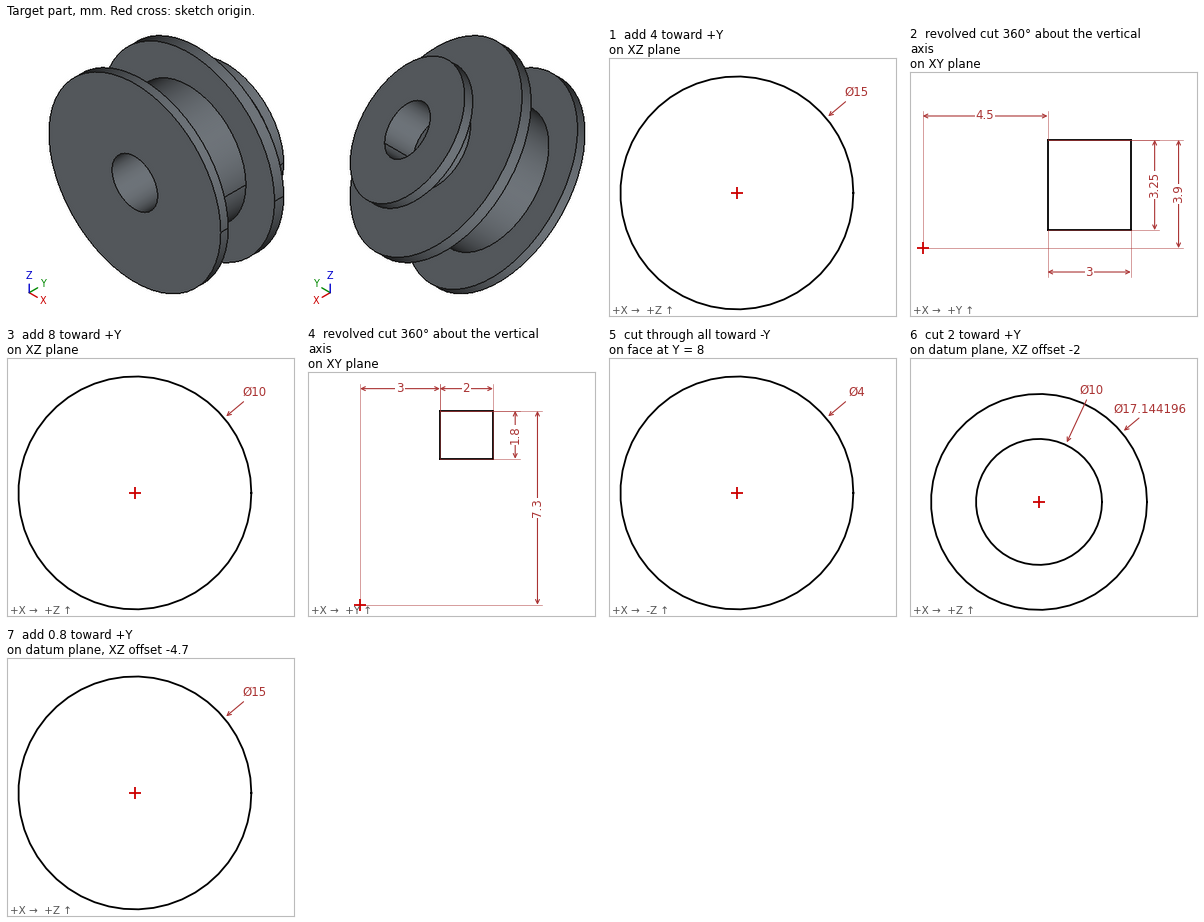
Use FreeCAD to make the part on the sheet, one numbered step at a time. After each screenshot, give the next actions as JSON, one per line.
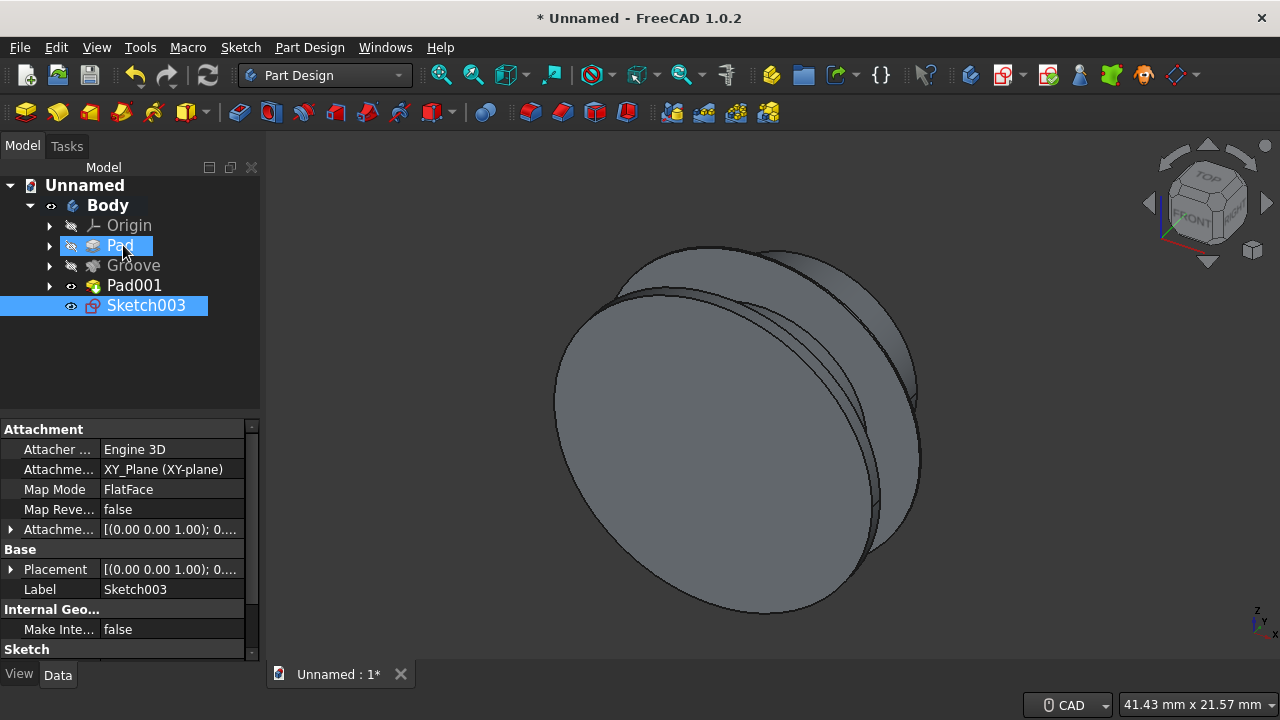
{"action": "left_click", "coordinate": [304, 112]}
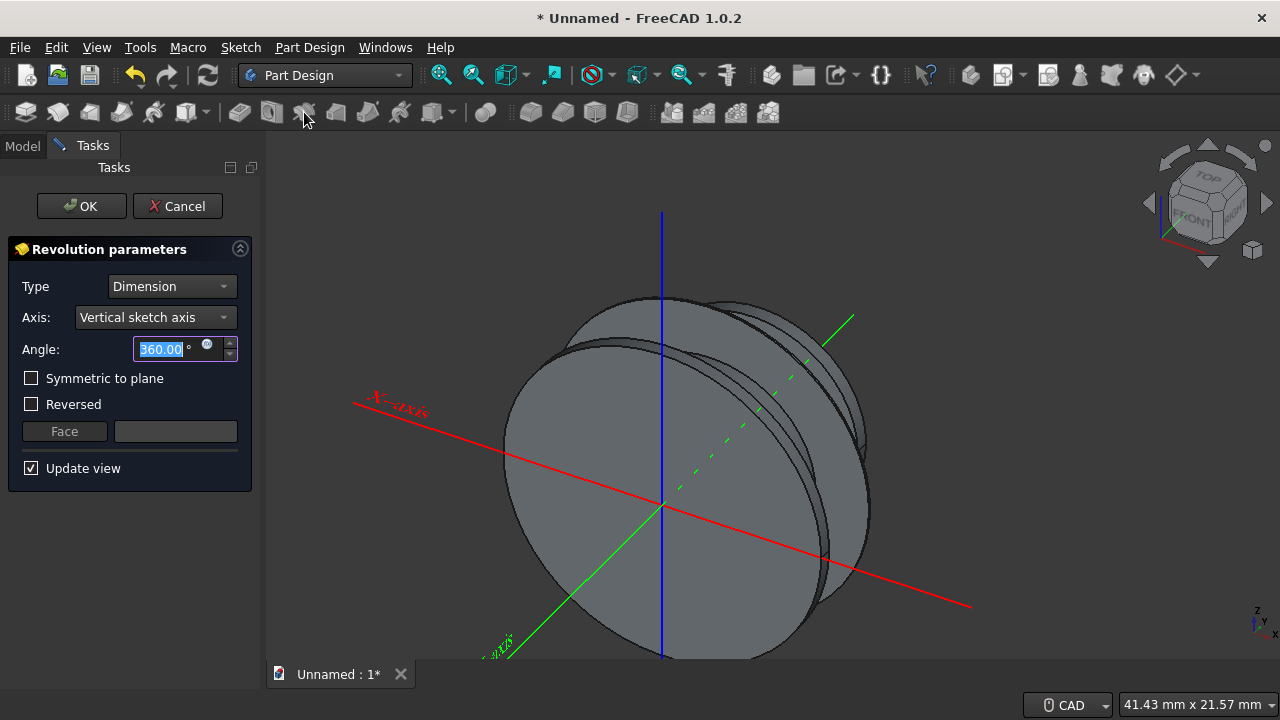
{"action": "left_click", "coordinate": [82, 206]}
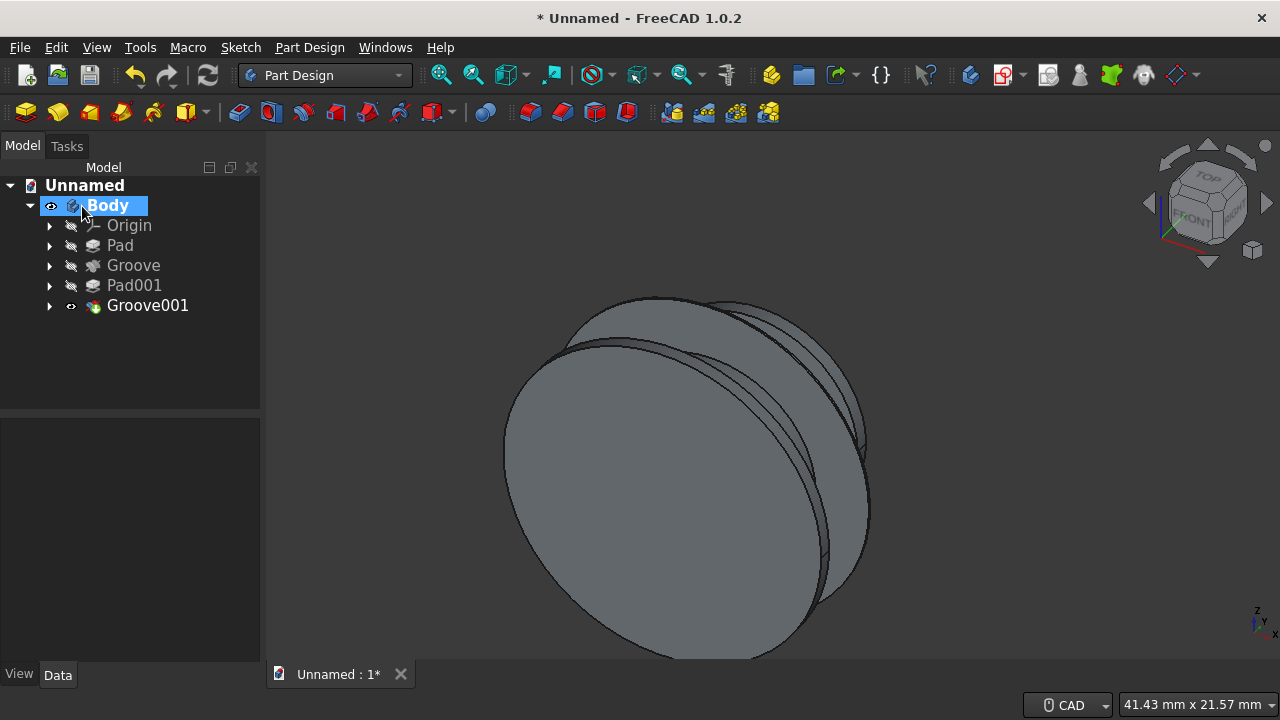
{"action": "left_click", "coordinate": [442, 76]}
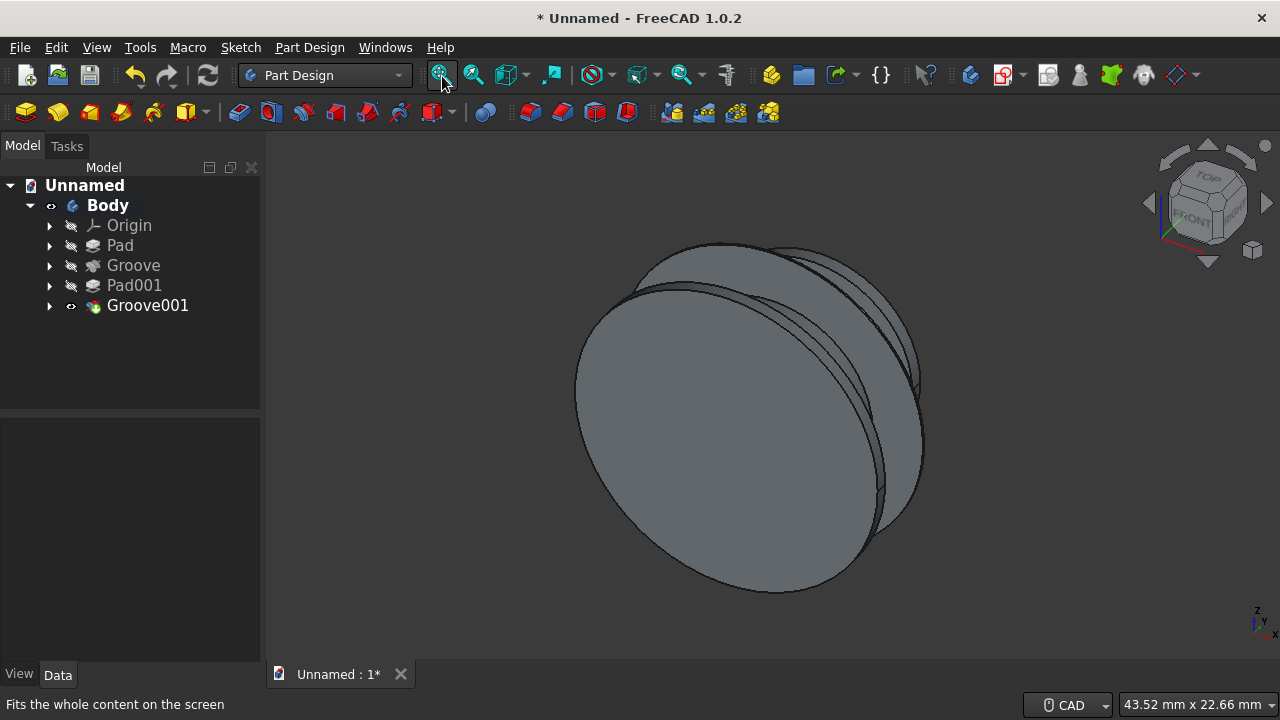
{"action": "key", "text": "4"}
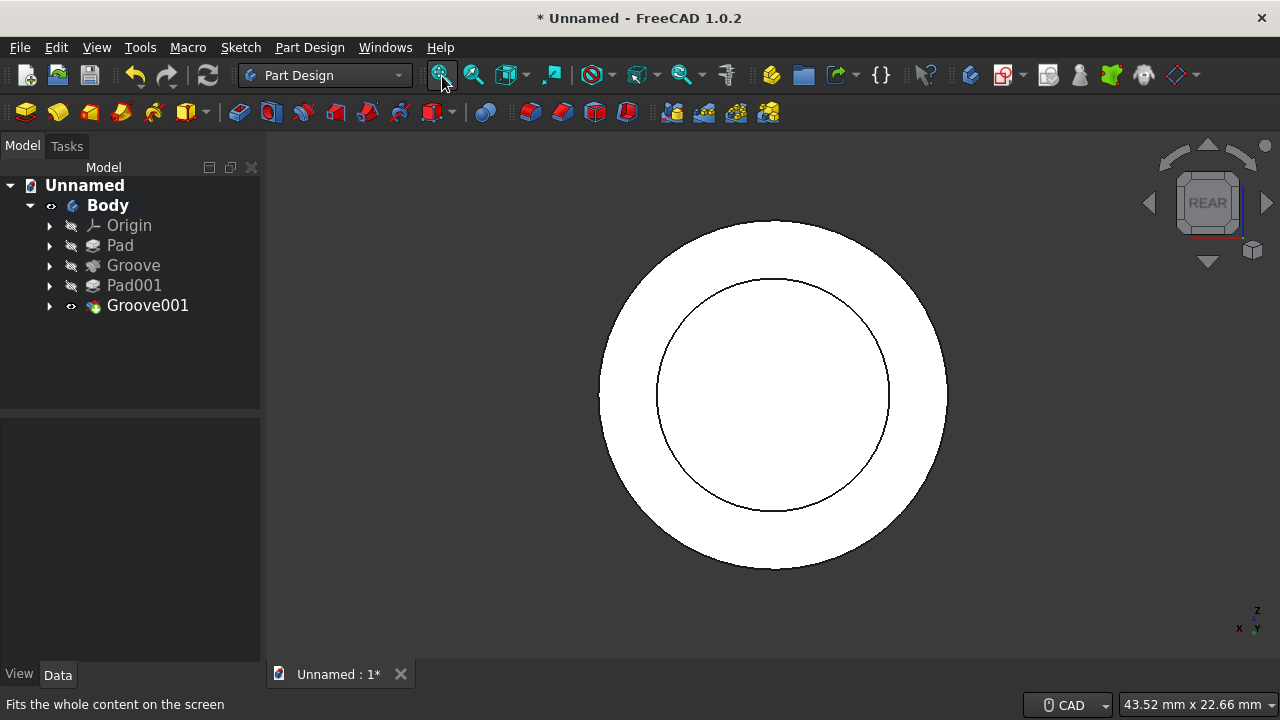
{"action": "left_click", "coordinate": [773, 394]}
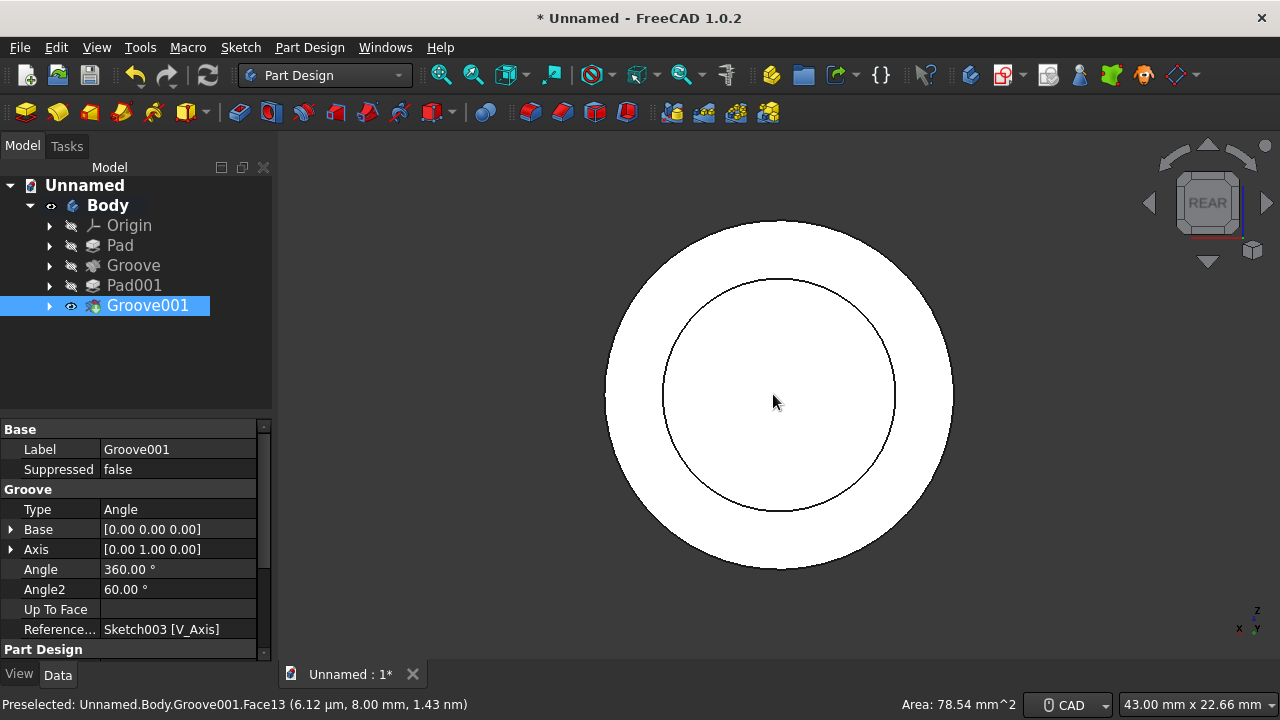
{"action": "left_click", "coordinate": [1004, 76]}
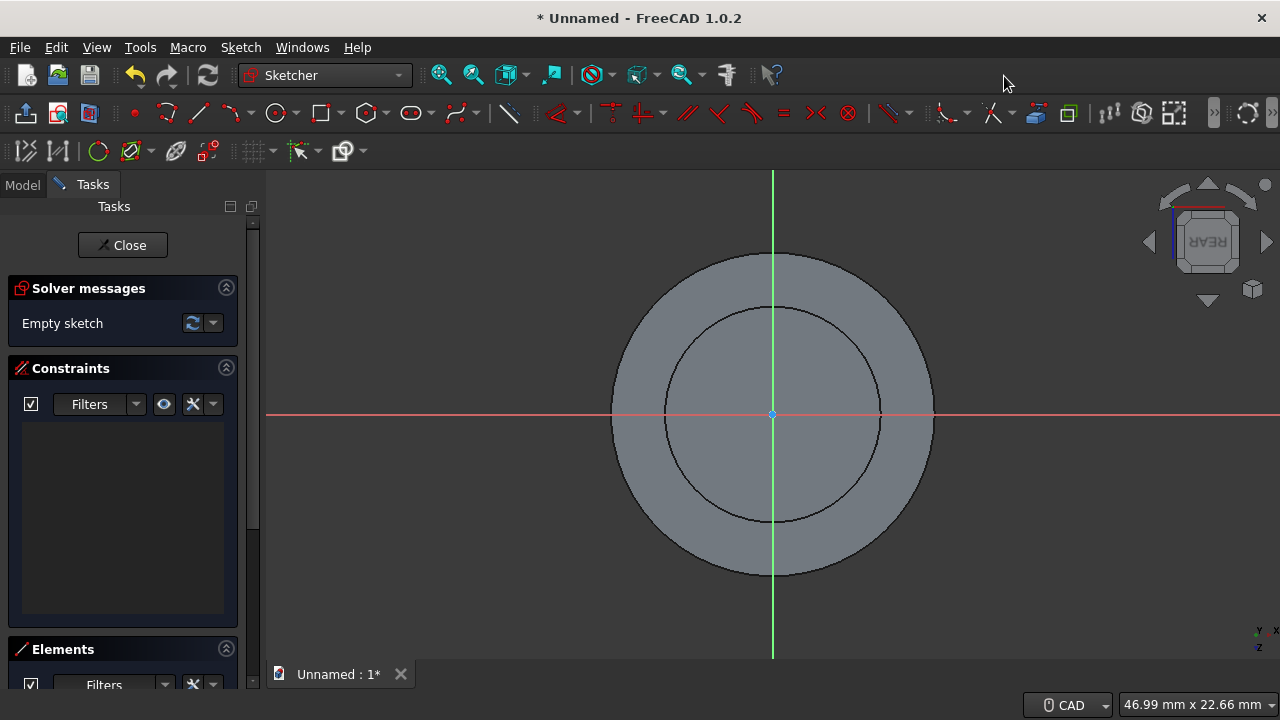
{"action": "scroll", "coordinate": [802, 414], "scroll_direction": "up", "scroll_amount": 6}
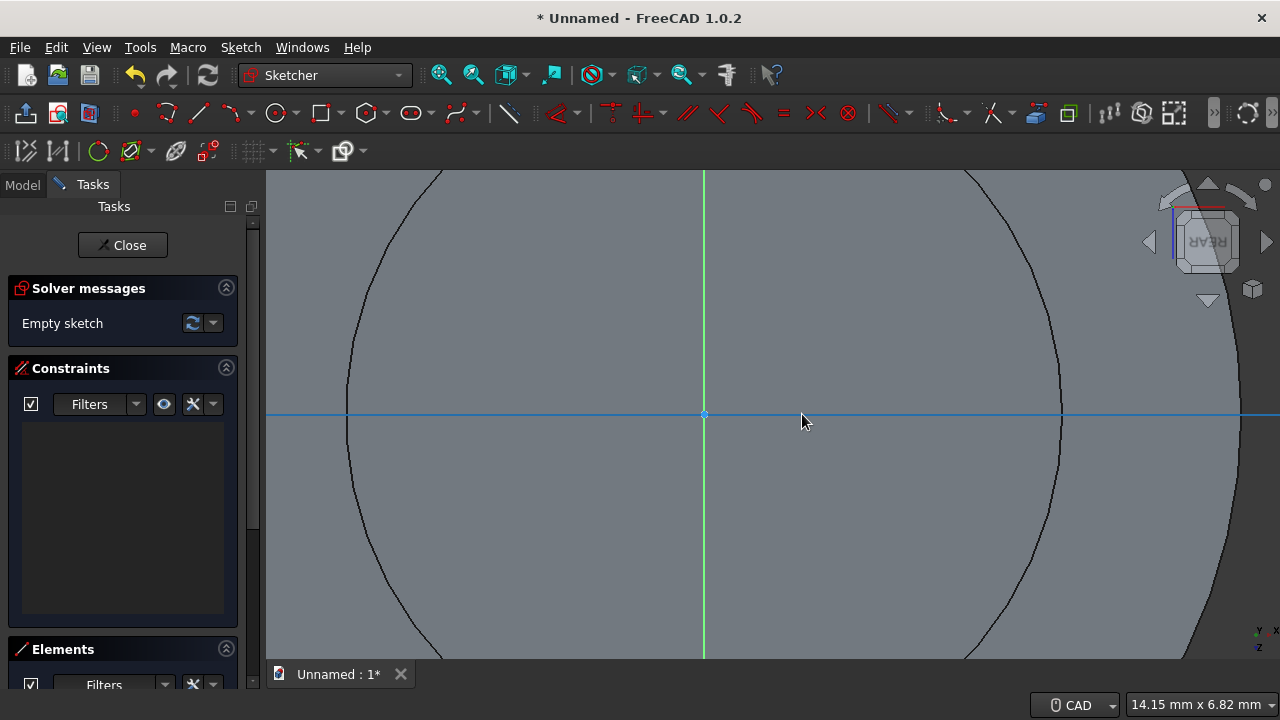
{"action": "left_click", "coordinate": [276, 114]}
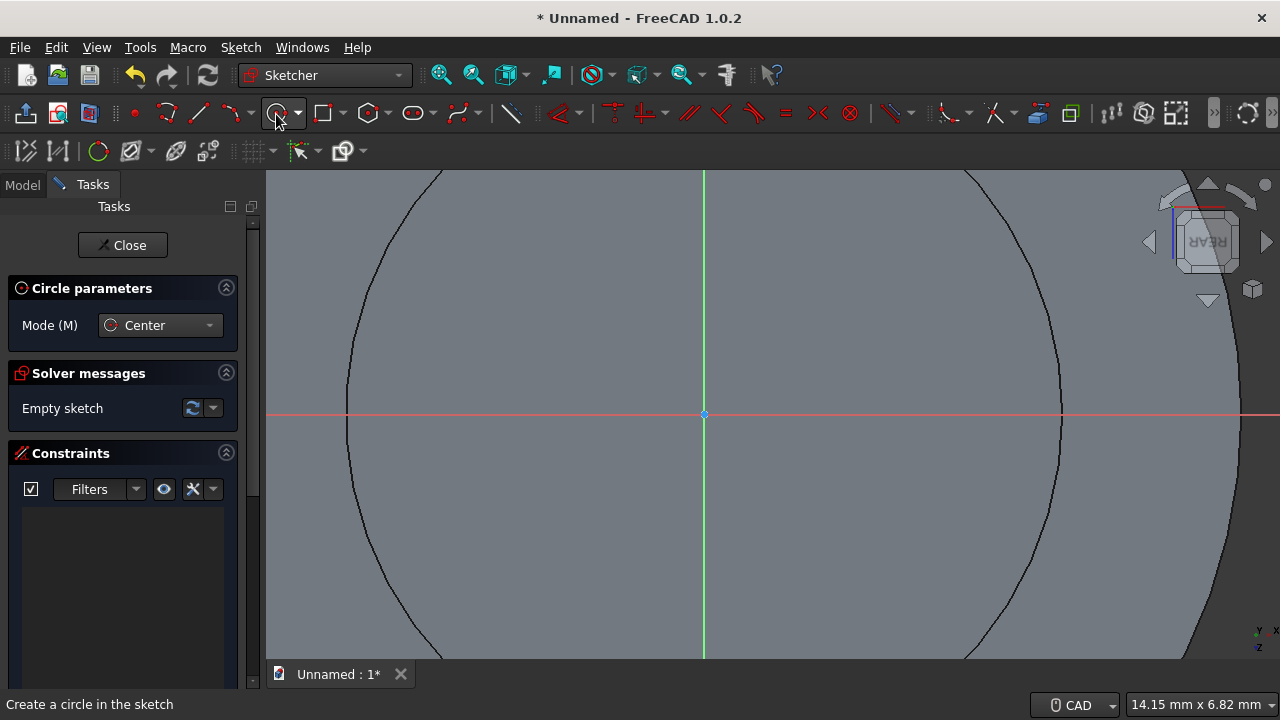
{"action": "left_click", "coordinate": [704, 414]}
{"action": "left_click", "coordinate": [805, 313]}
{"action": "key", "text": "Escape"}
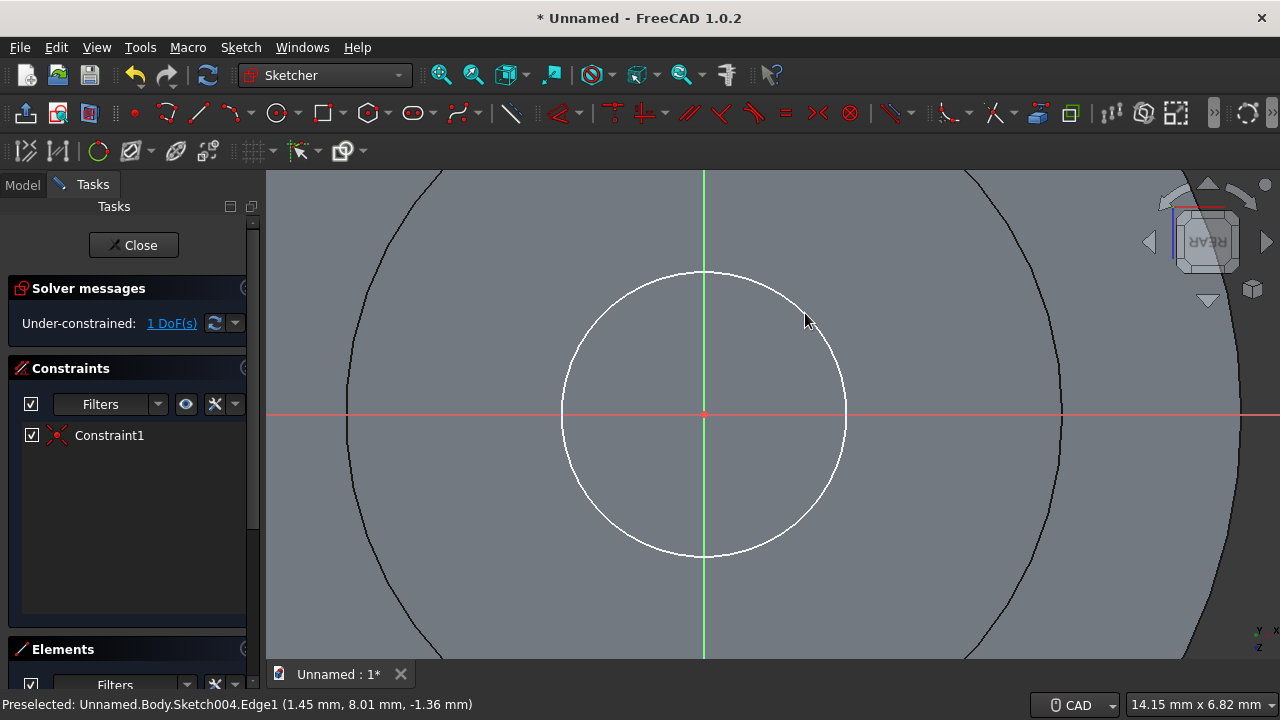
{"action": "left_click", "coordinate": [558, 114]}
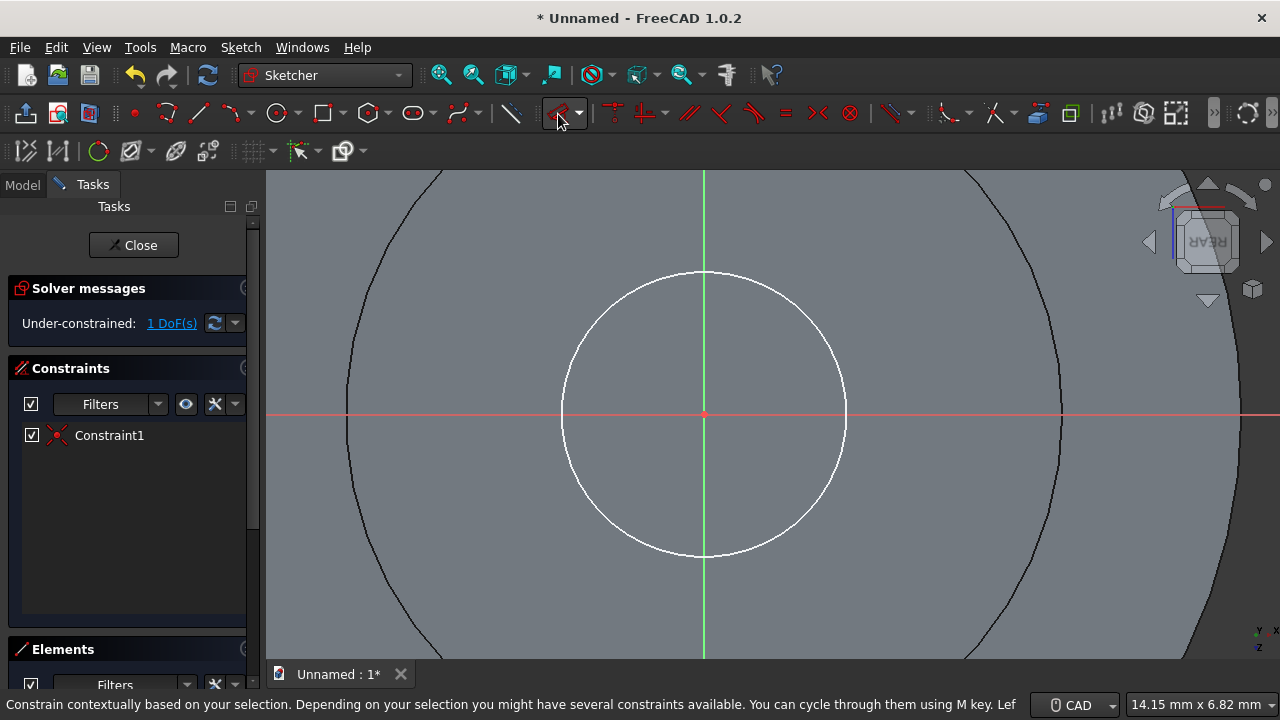
{"action": "left_click", "coordinate": [804, 313]}
{"action": "left_click", "coordinate": [826, 290]}